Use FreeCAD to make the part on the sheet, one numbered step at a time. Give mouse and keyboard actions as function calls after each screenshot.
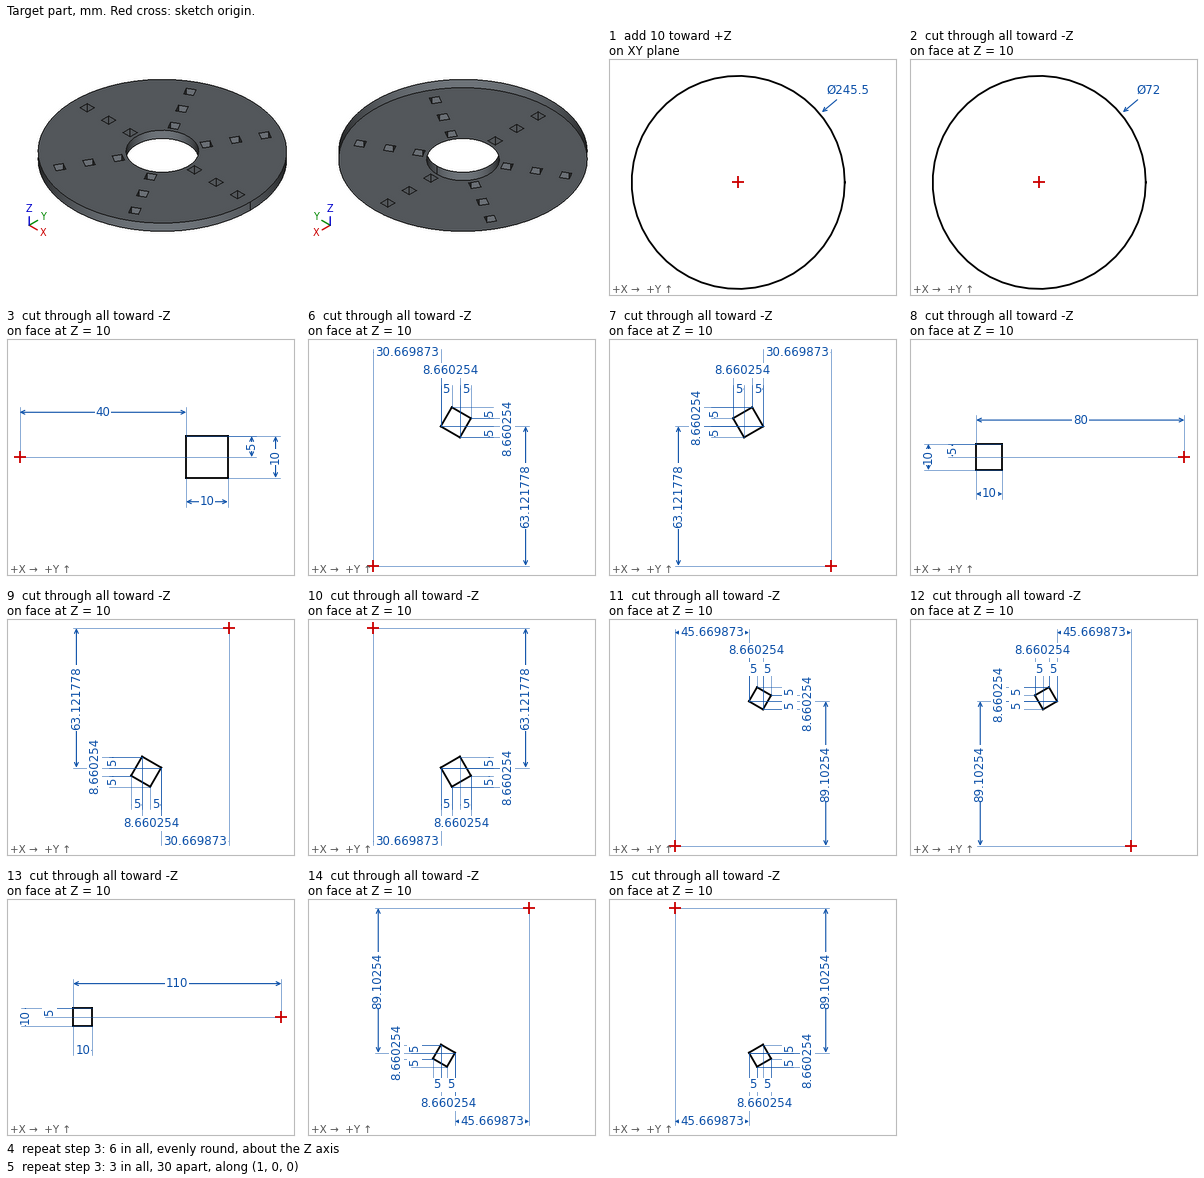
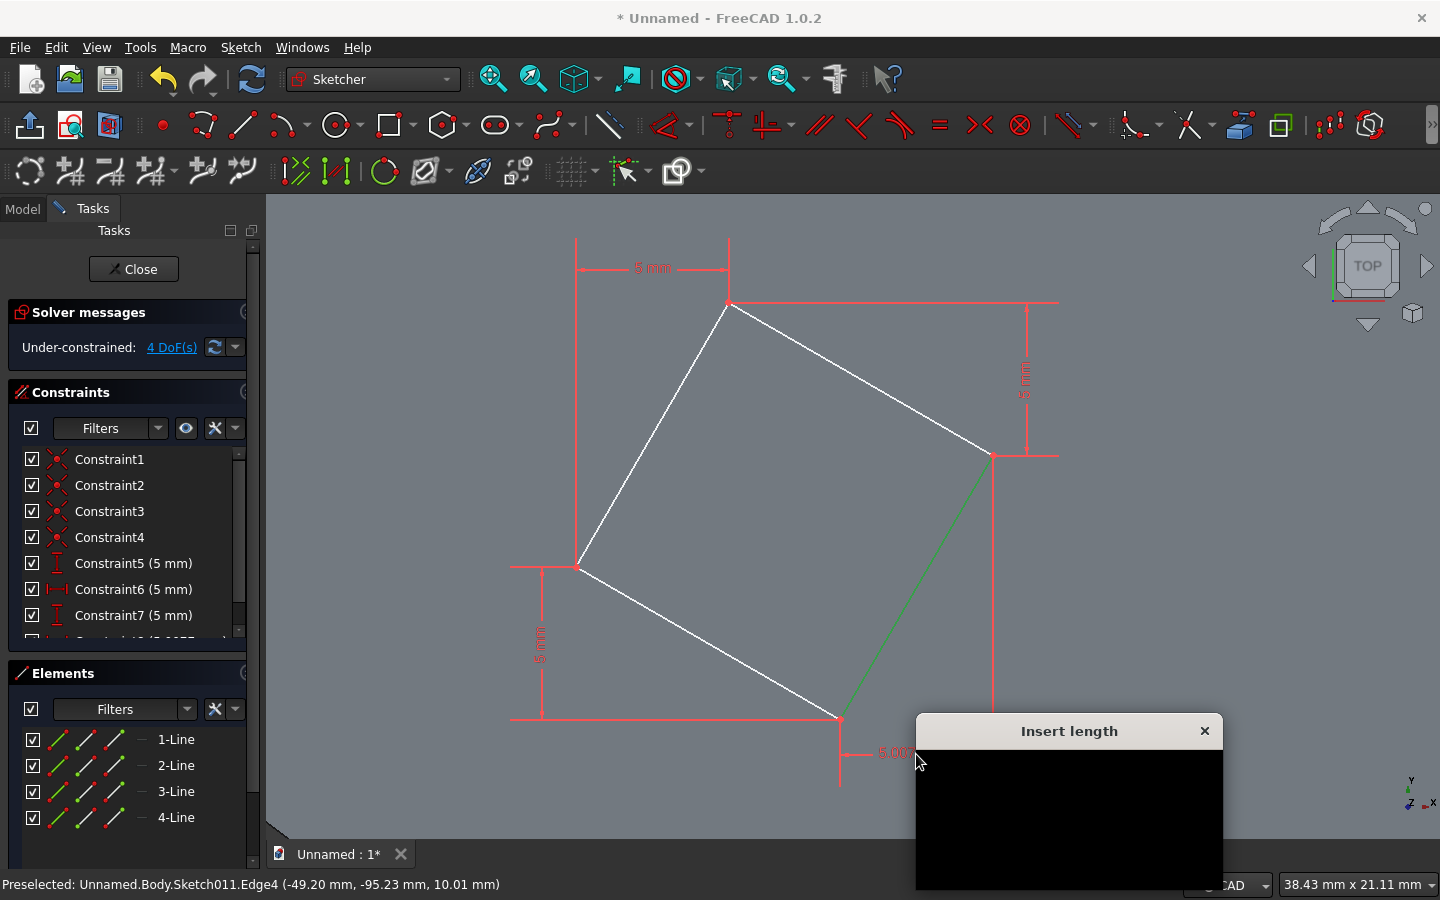
text(5)
key(Return)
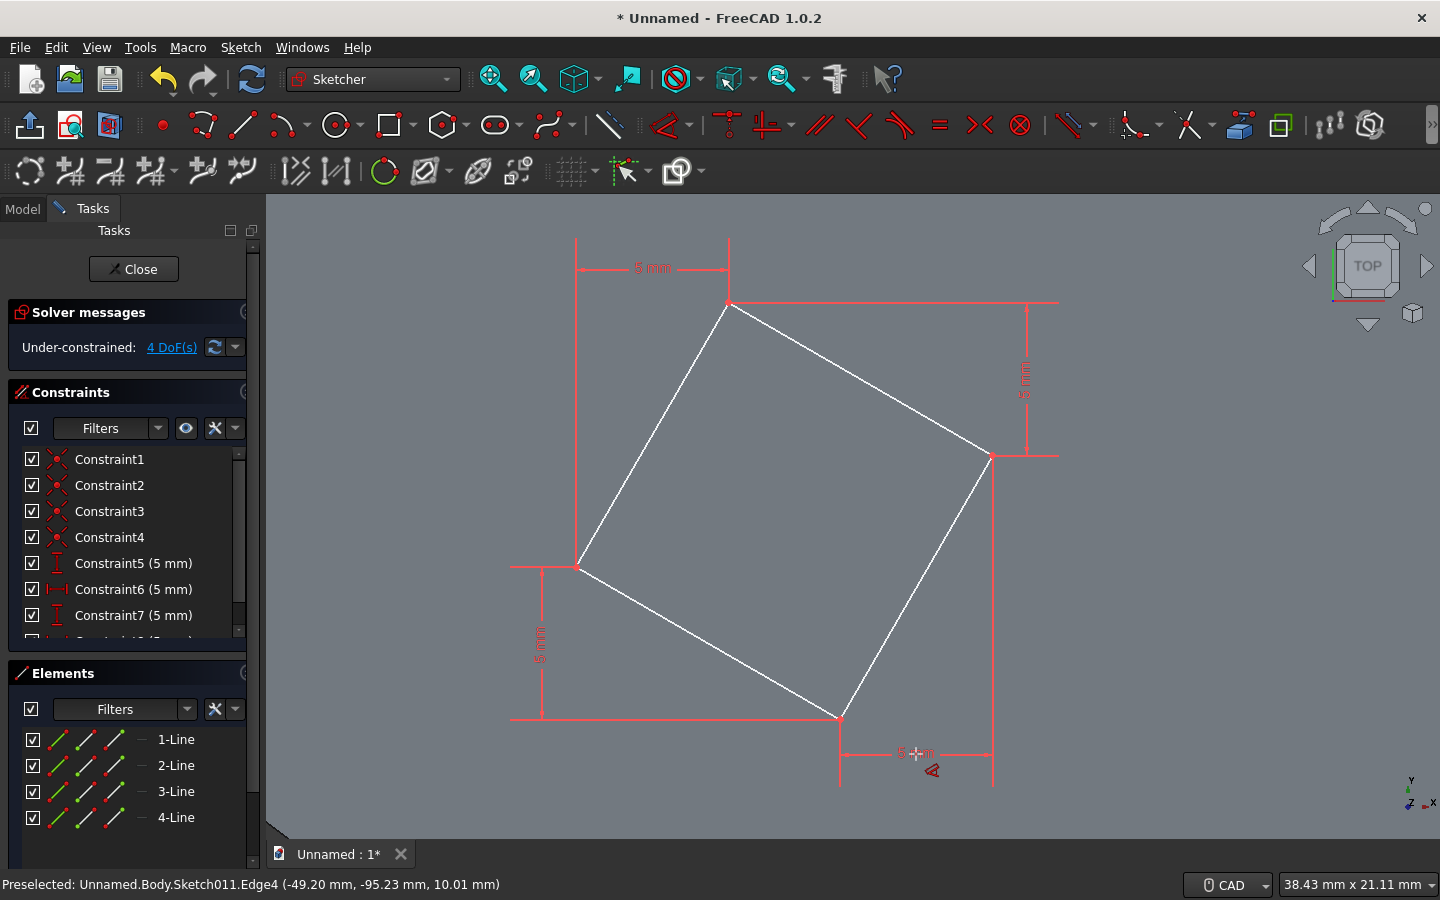
click(993, 456)
click(959, 339)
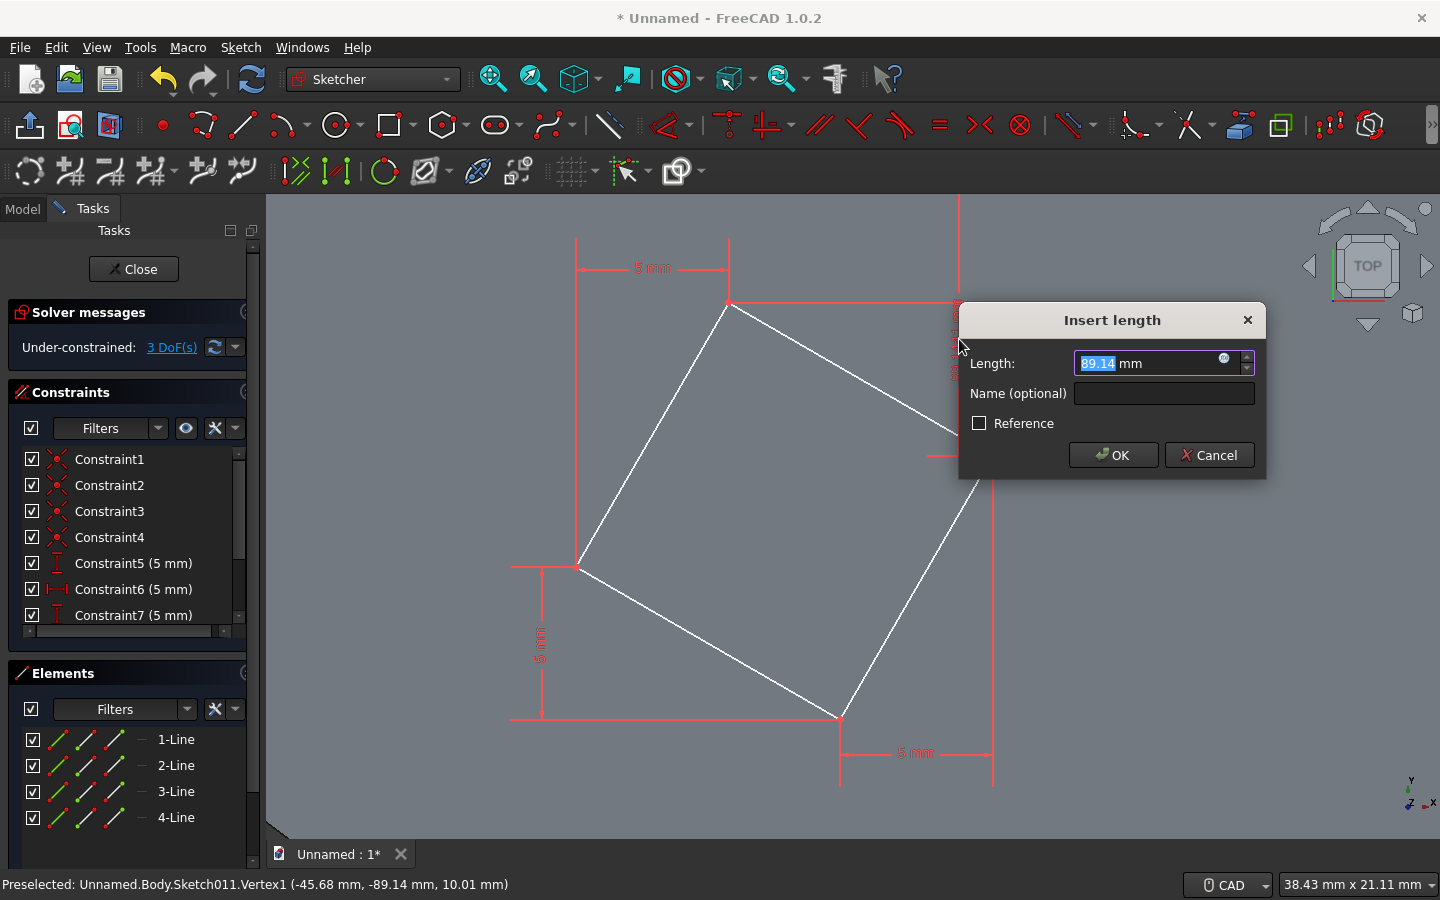
text(89.10254)
key(Return)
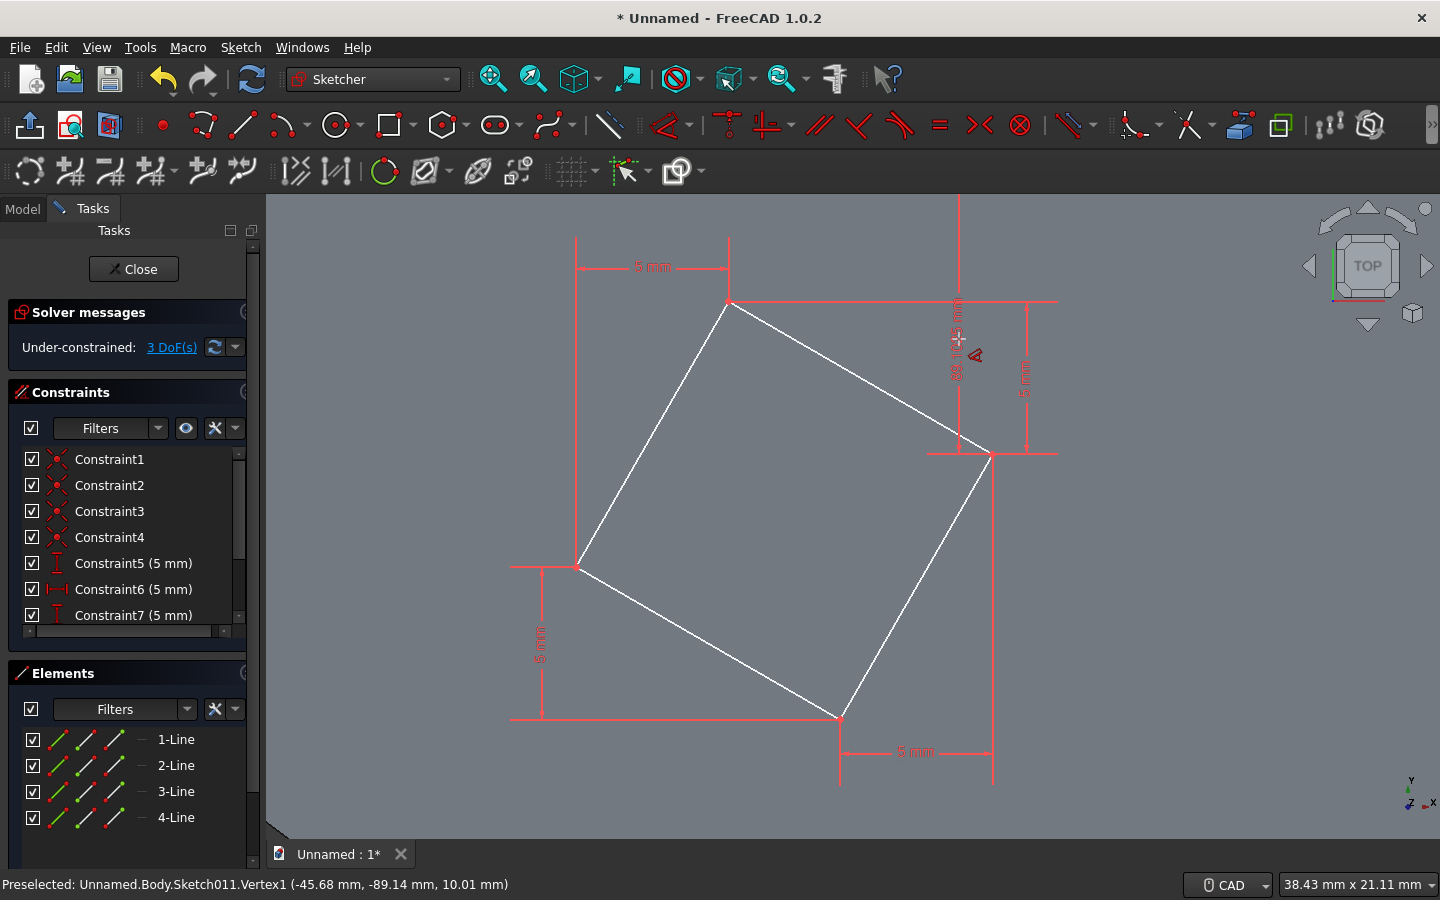
click(914, 409)
click(861, 268)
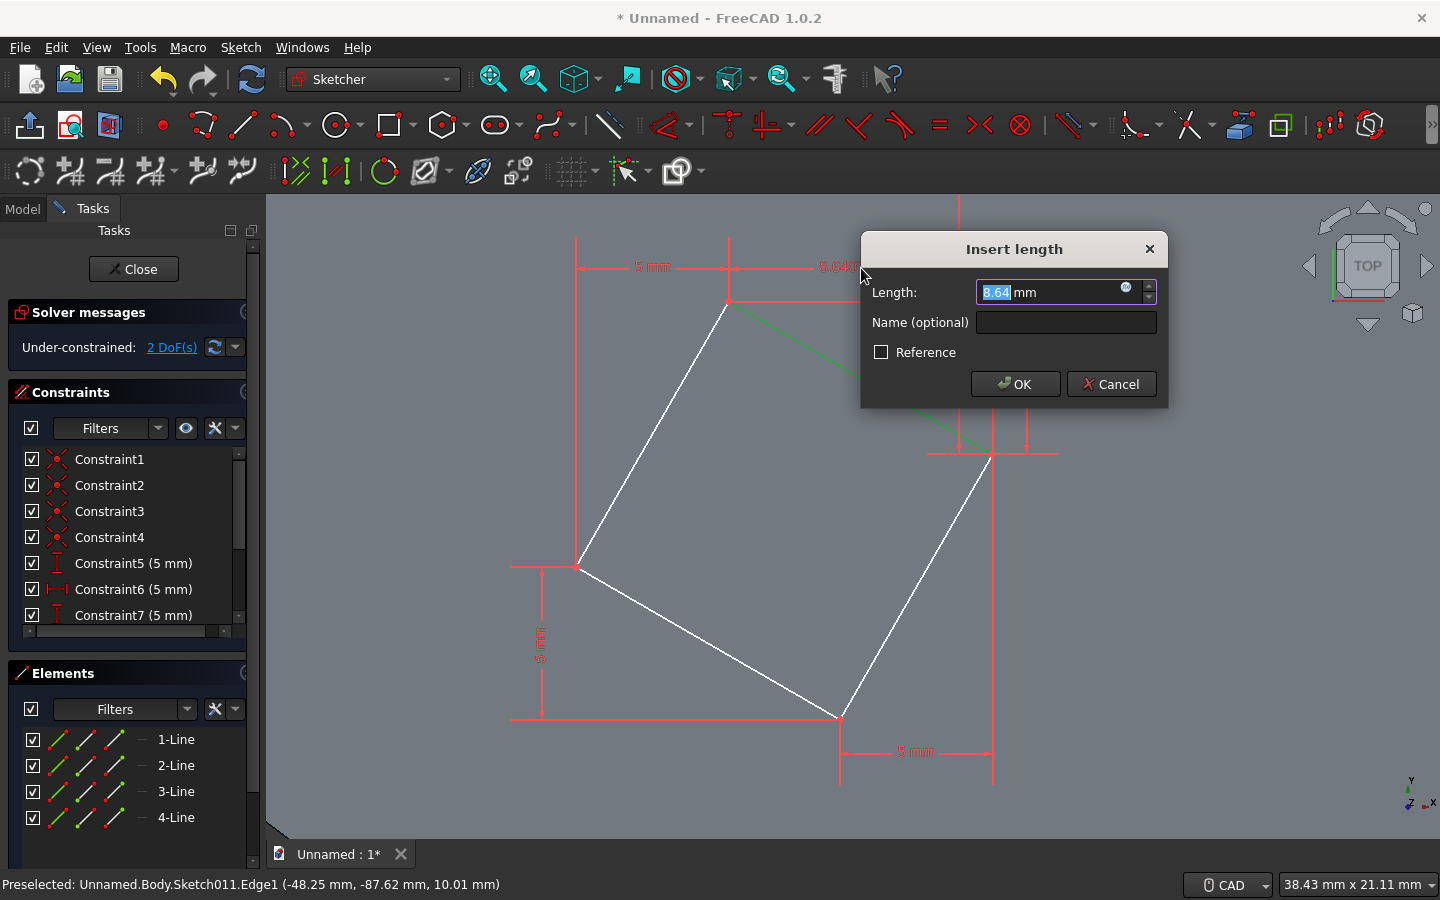
text(8.660254)
key(Return)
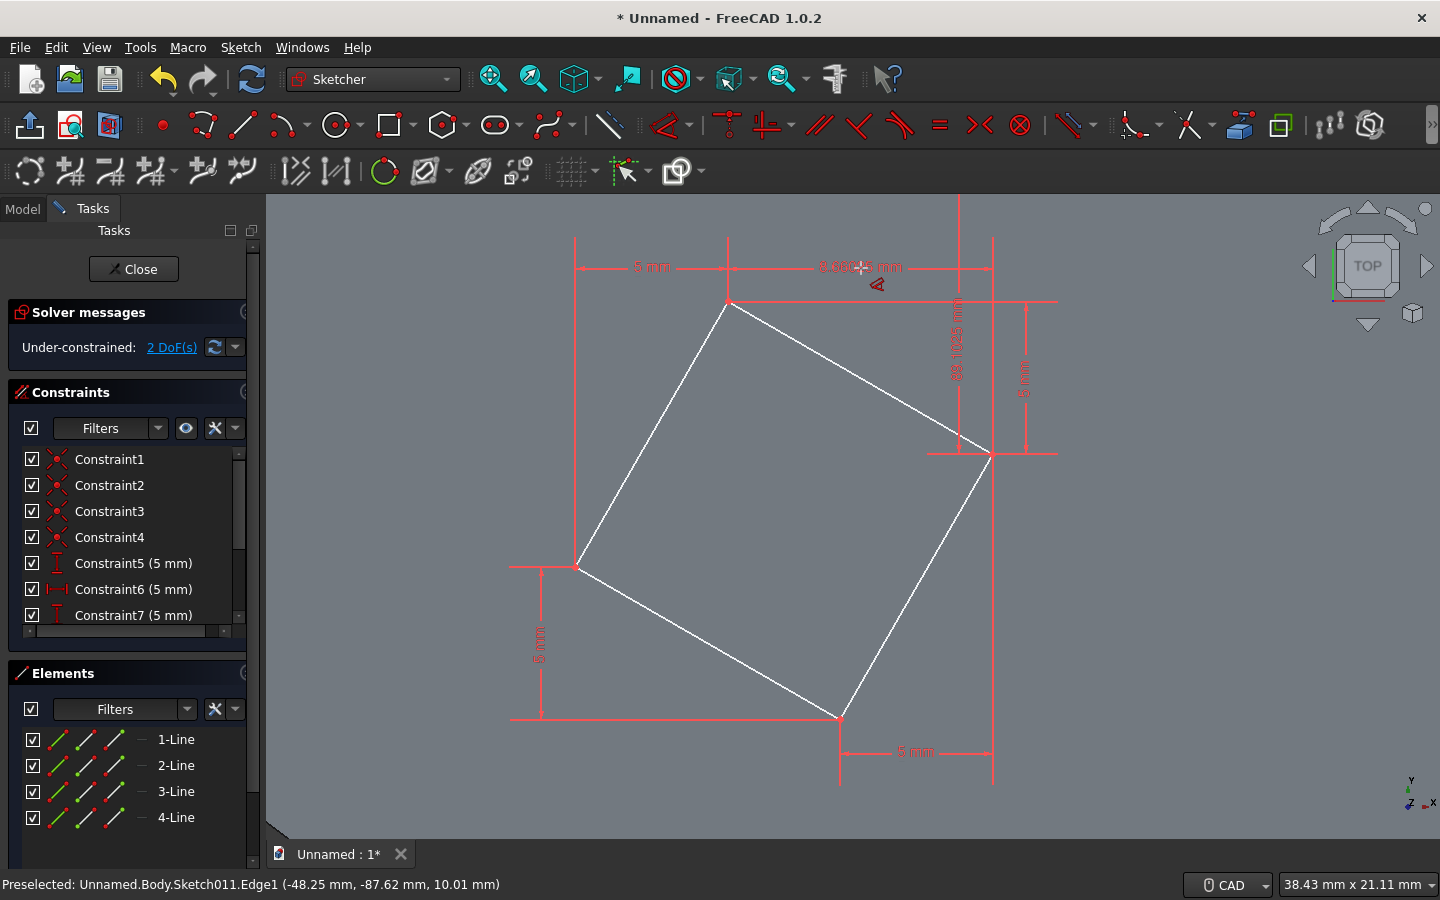
click(682, 381)
click(541, 434)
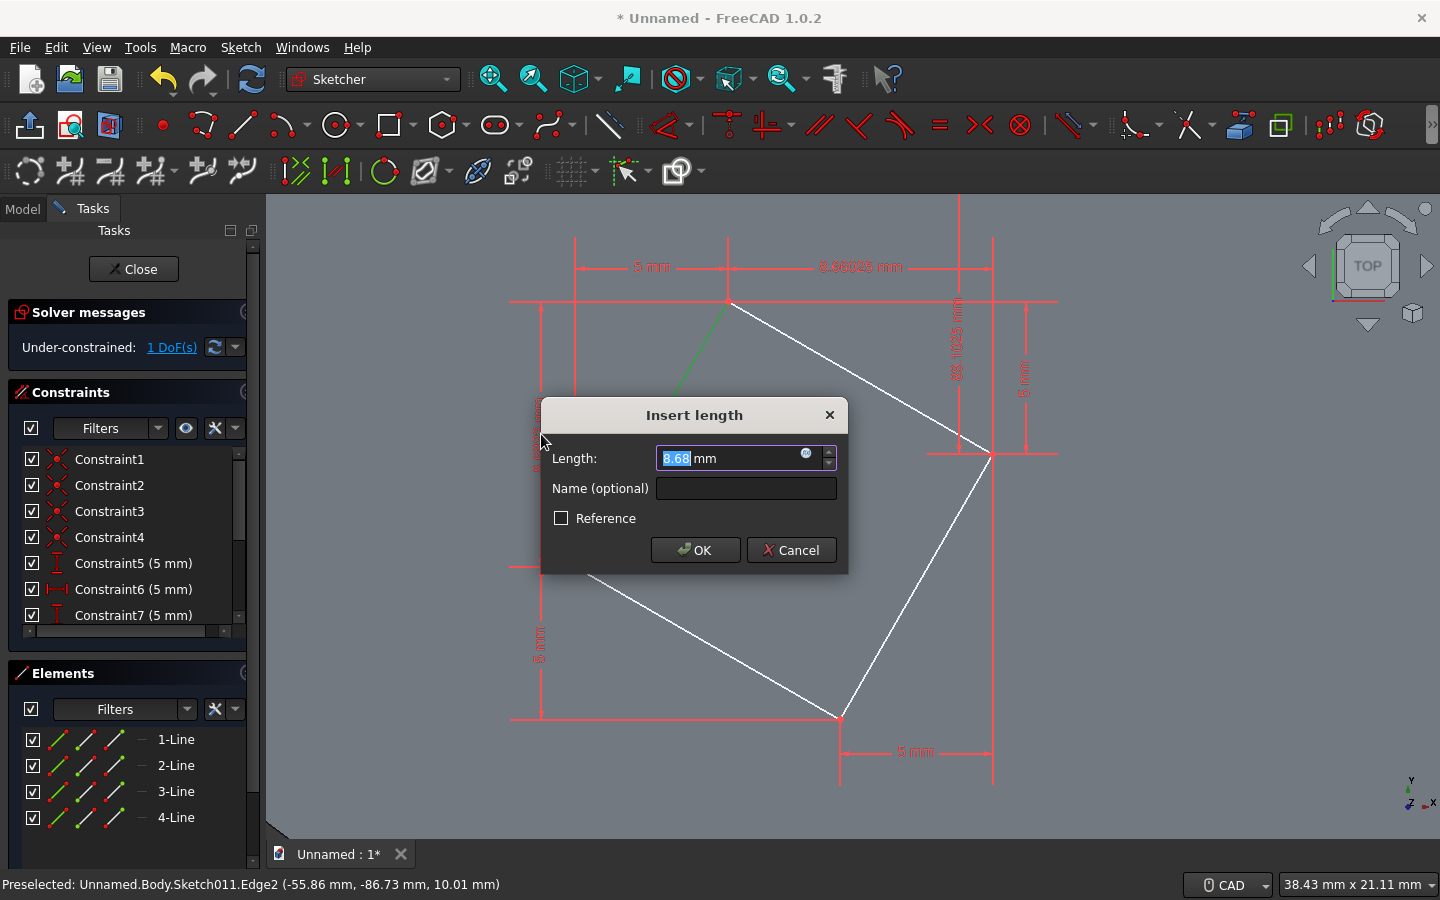
text(8.660254)
key(Return)